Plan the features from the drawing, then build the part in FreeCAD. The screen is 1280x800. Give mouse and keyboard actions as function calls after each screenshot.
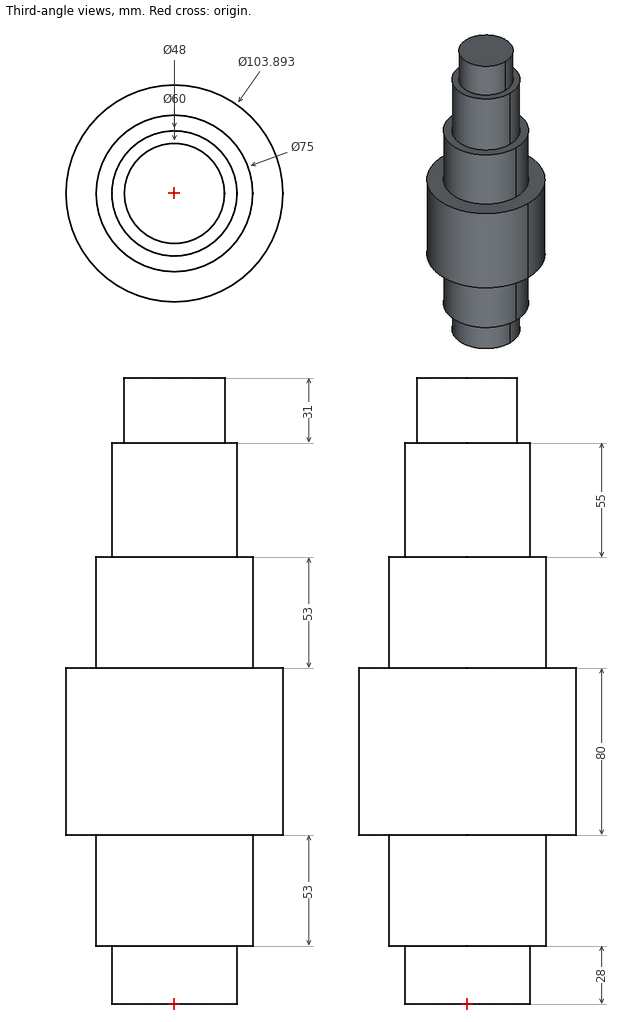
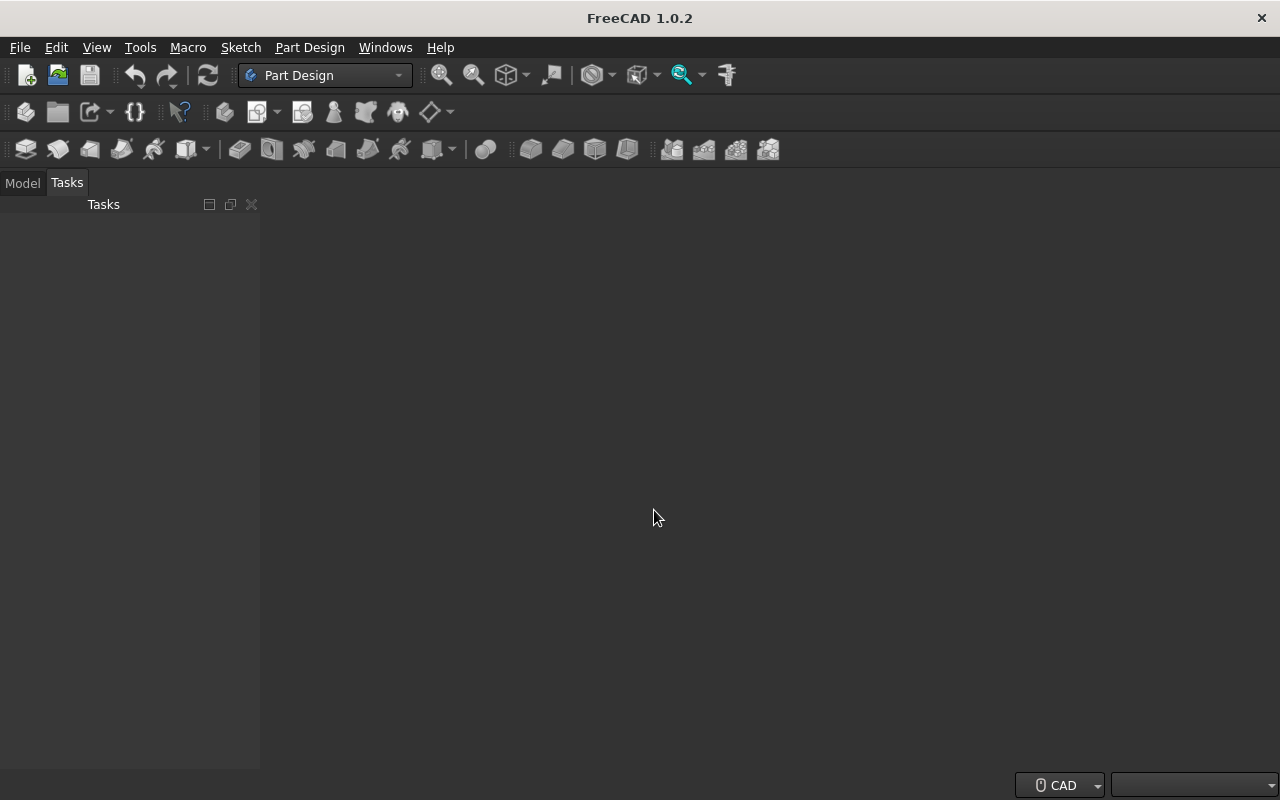
click(26, 76)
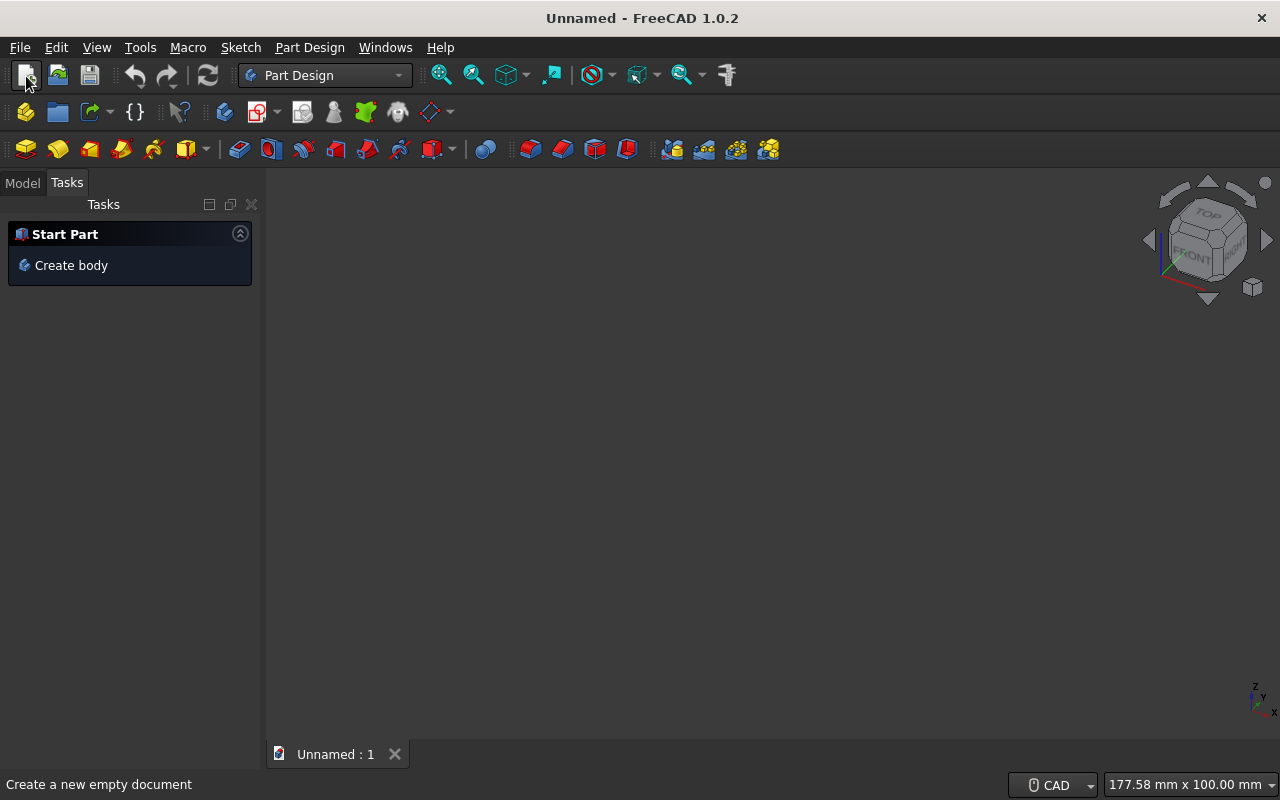
click(258, 112)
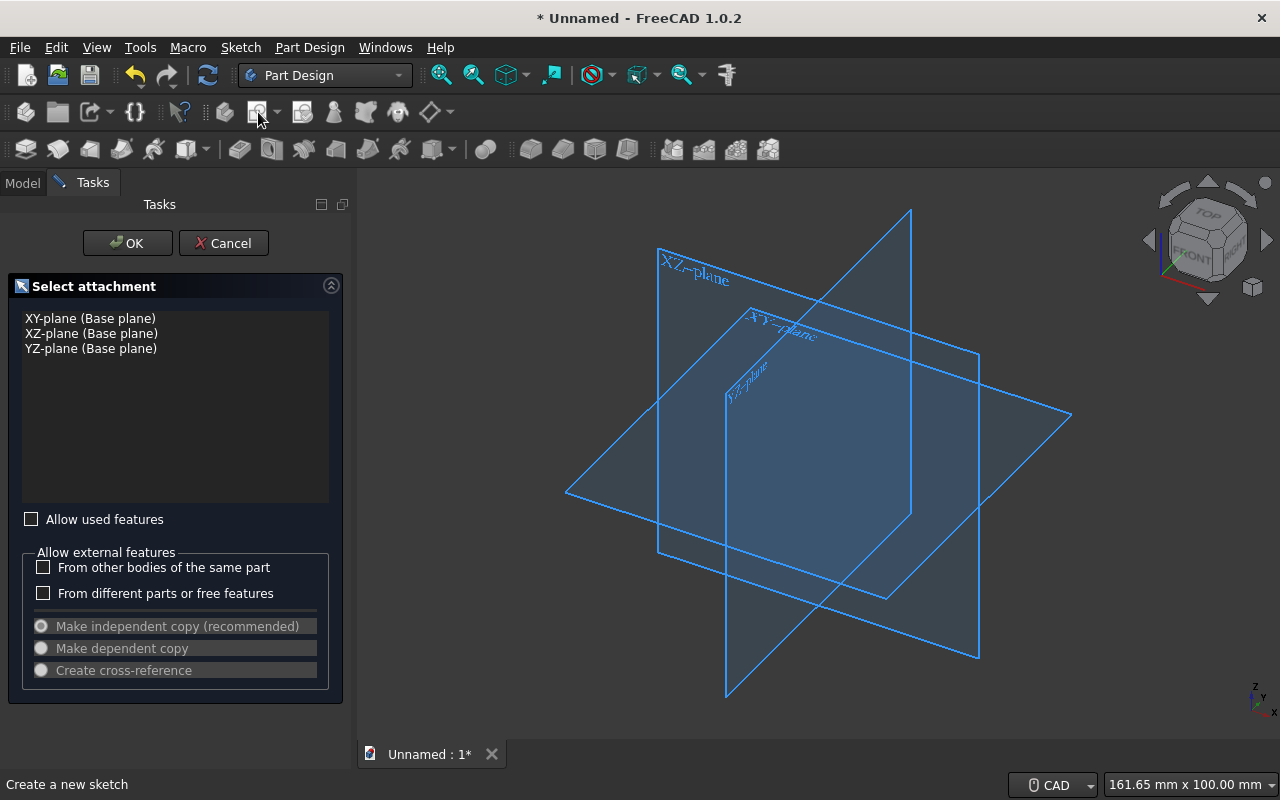
click(82, 318)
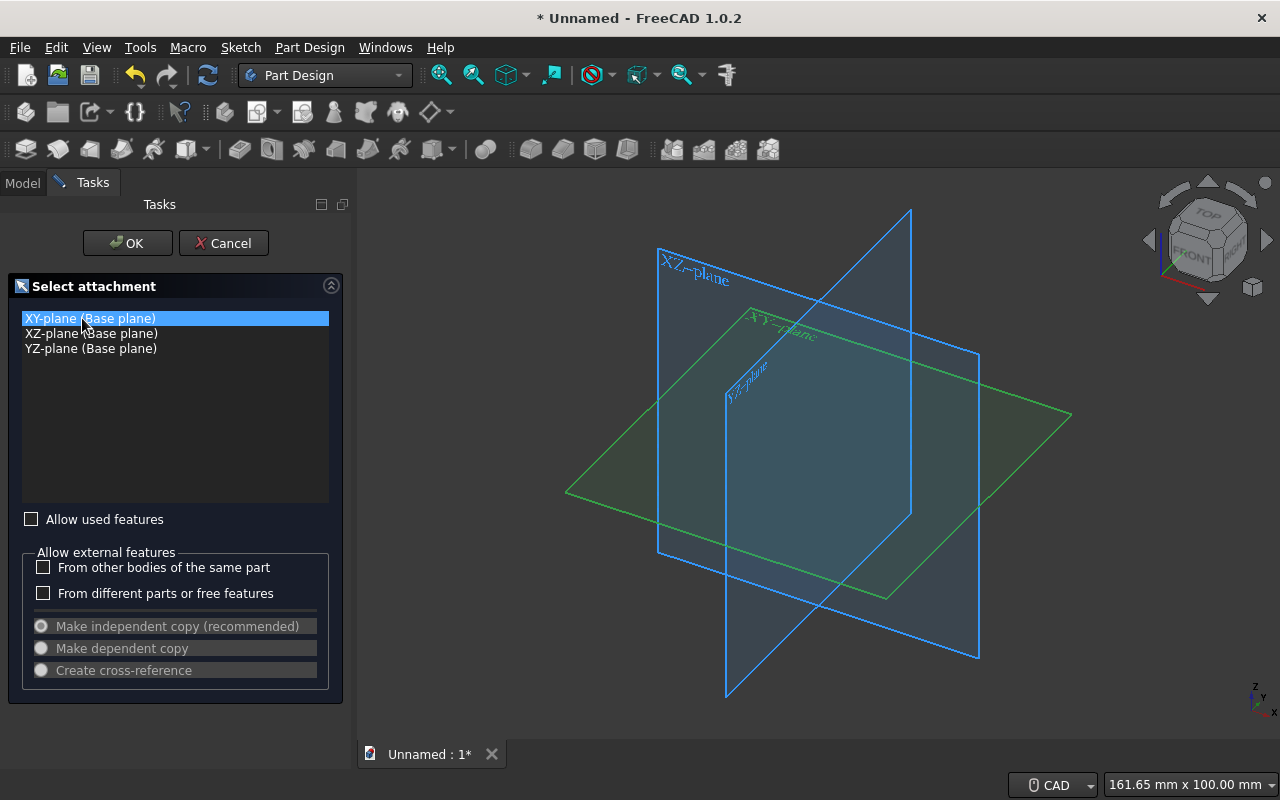
click(128, 243)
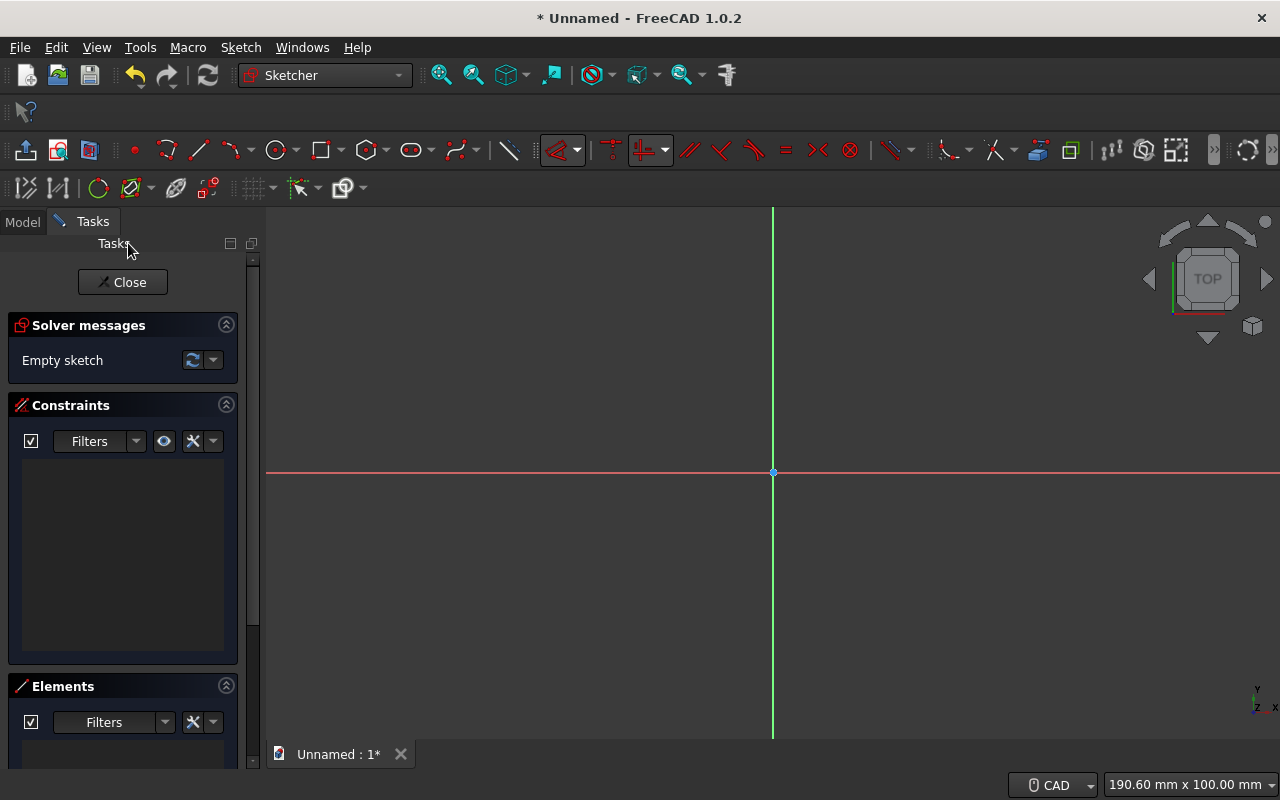
click(276, 150)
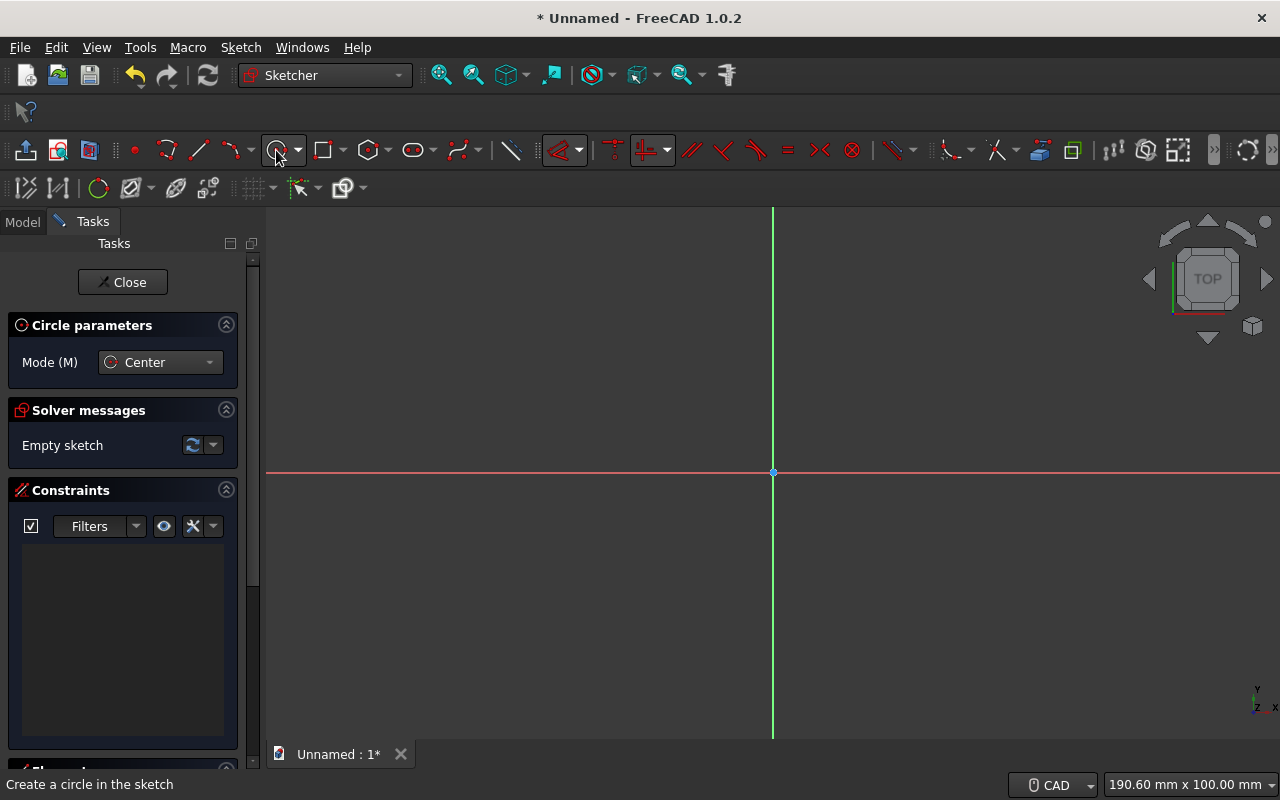
click(773, 473)
move(886, 360)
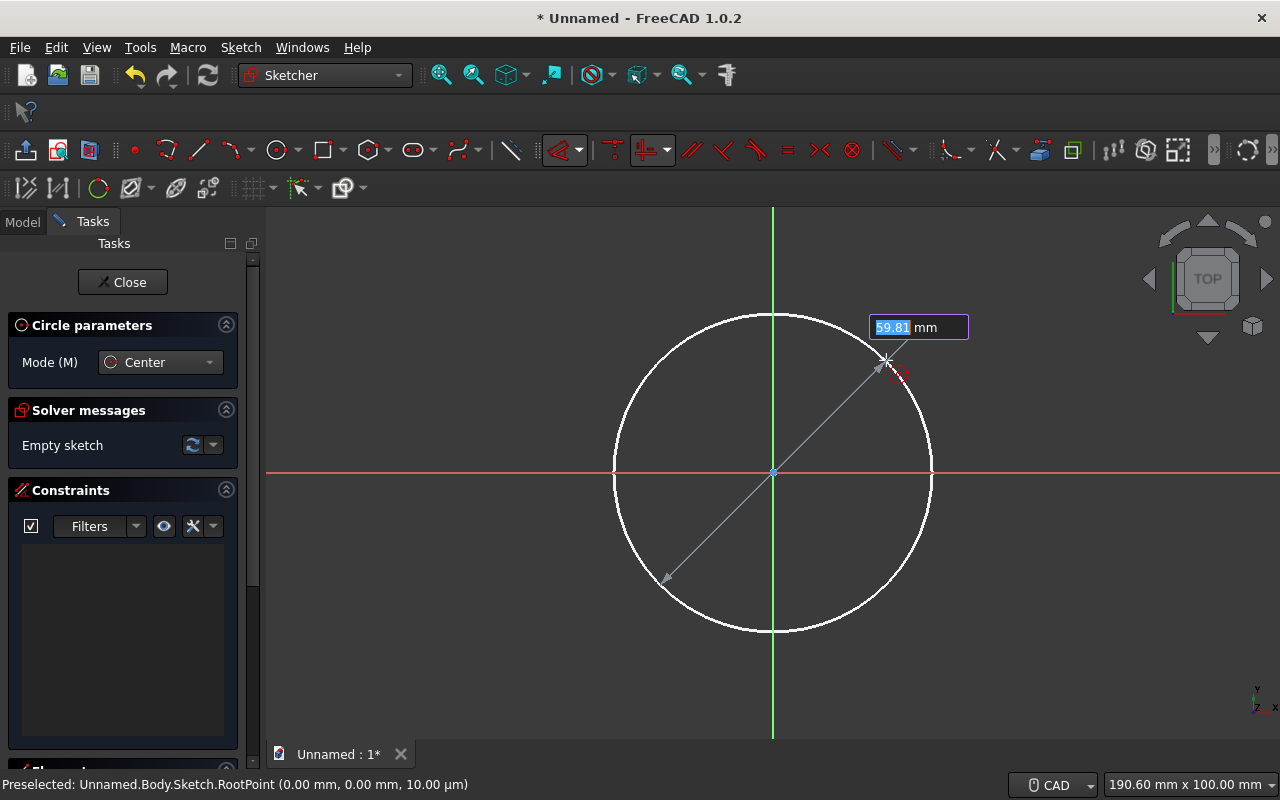
text(60)
key(Return)
key(Escape)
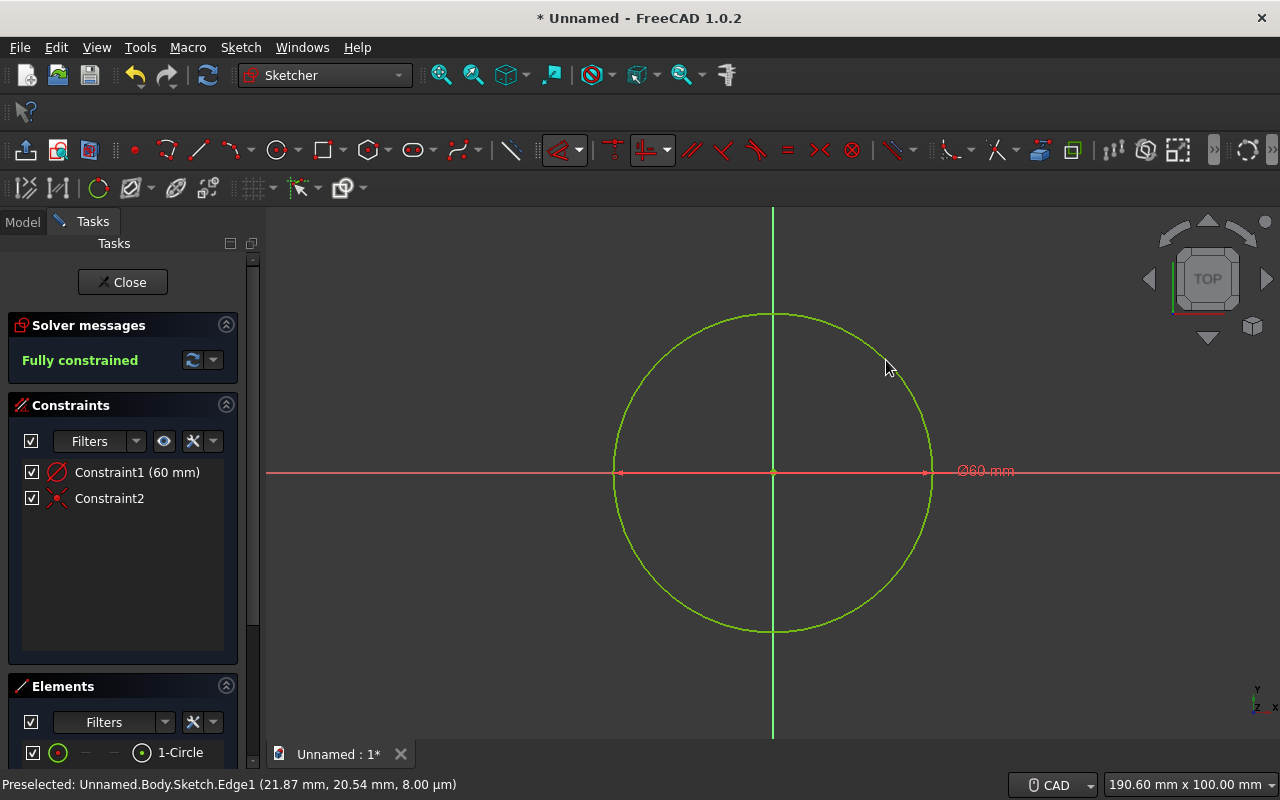
click(123, 282)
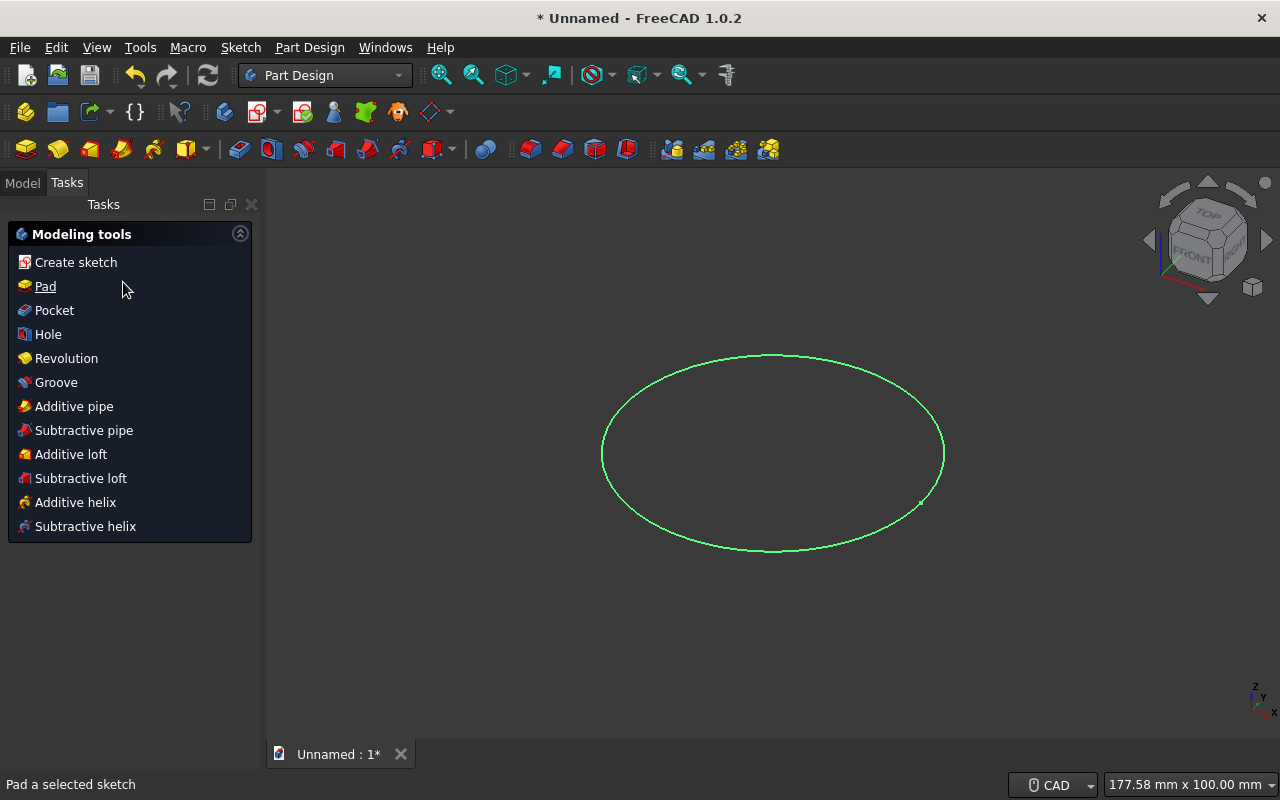
click(26, 150)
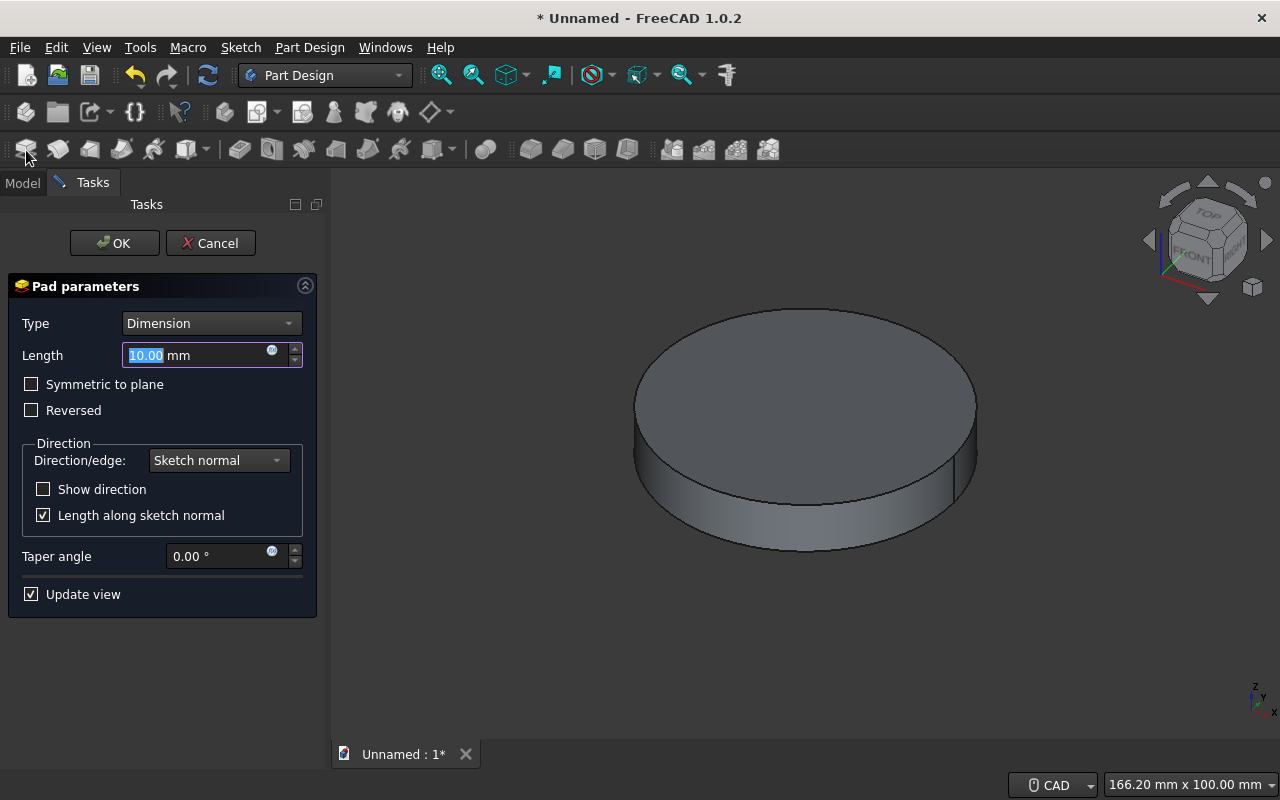
text(28)
key(Tab)